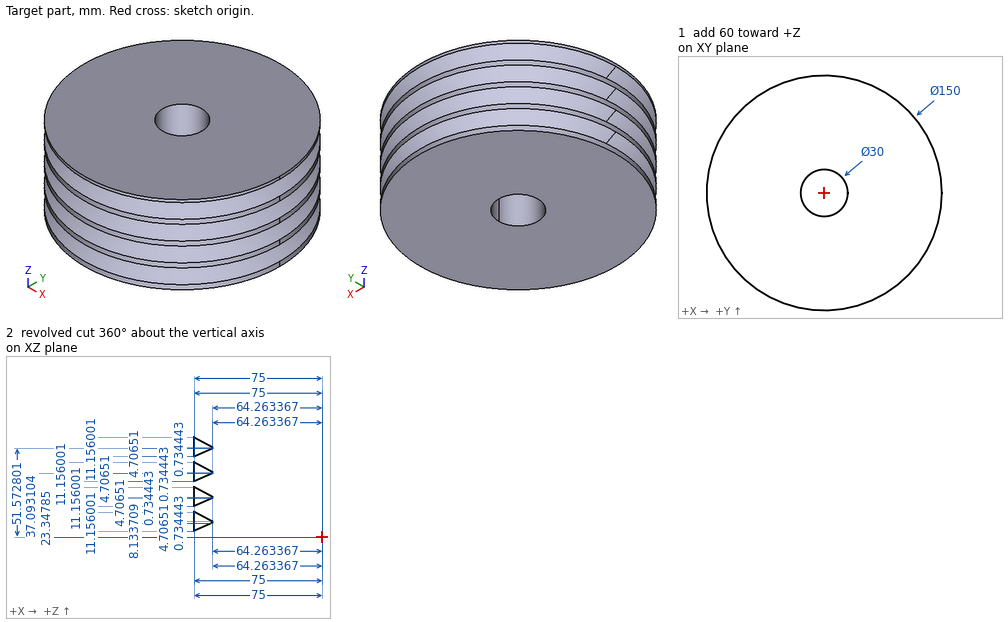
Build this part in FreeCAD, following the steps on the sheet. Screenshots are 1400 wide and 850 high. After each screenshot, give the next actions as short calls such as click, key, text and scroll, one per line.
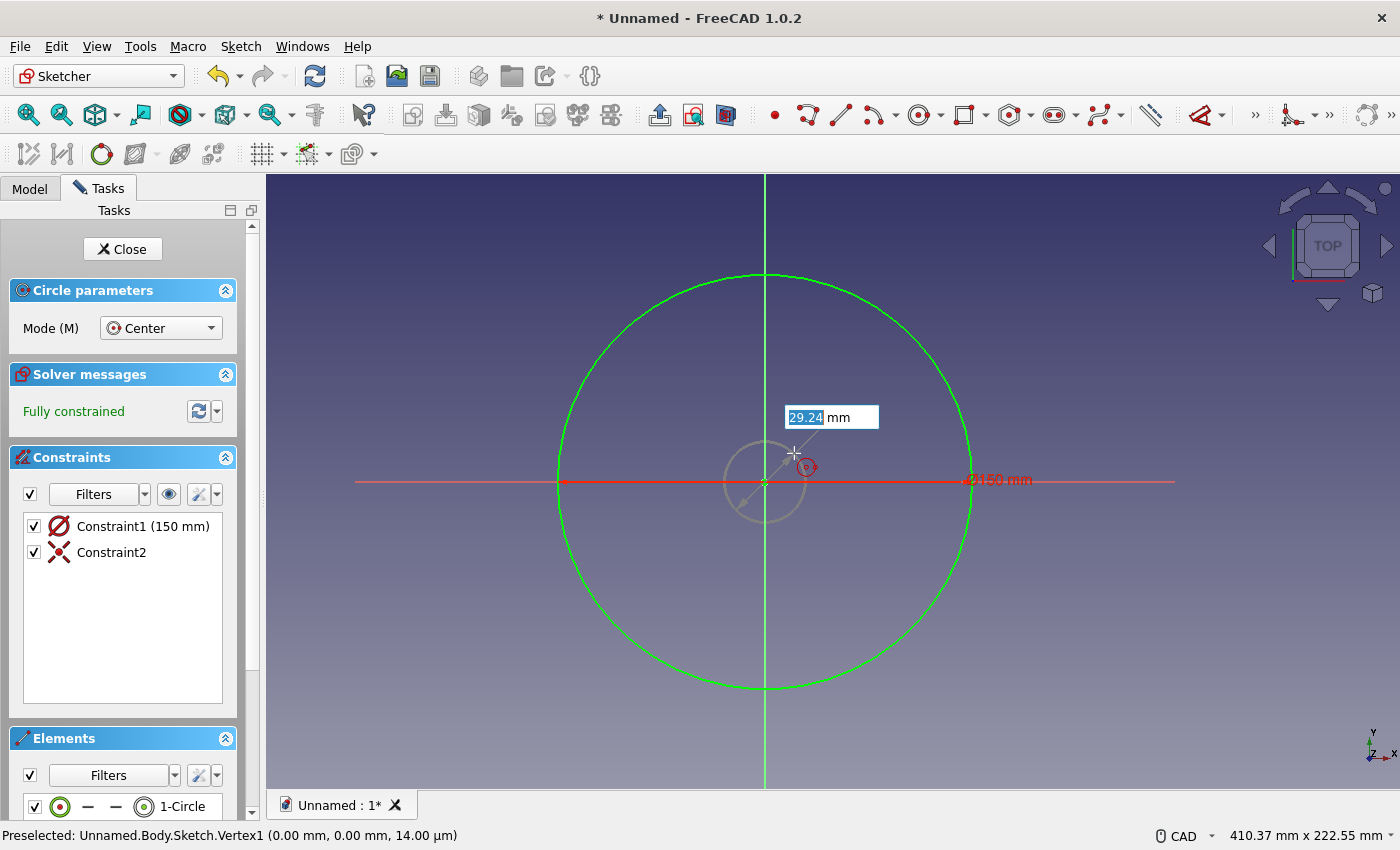
text(30)
key(Return)
key(Escape)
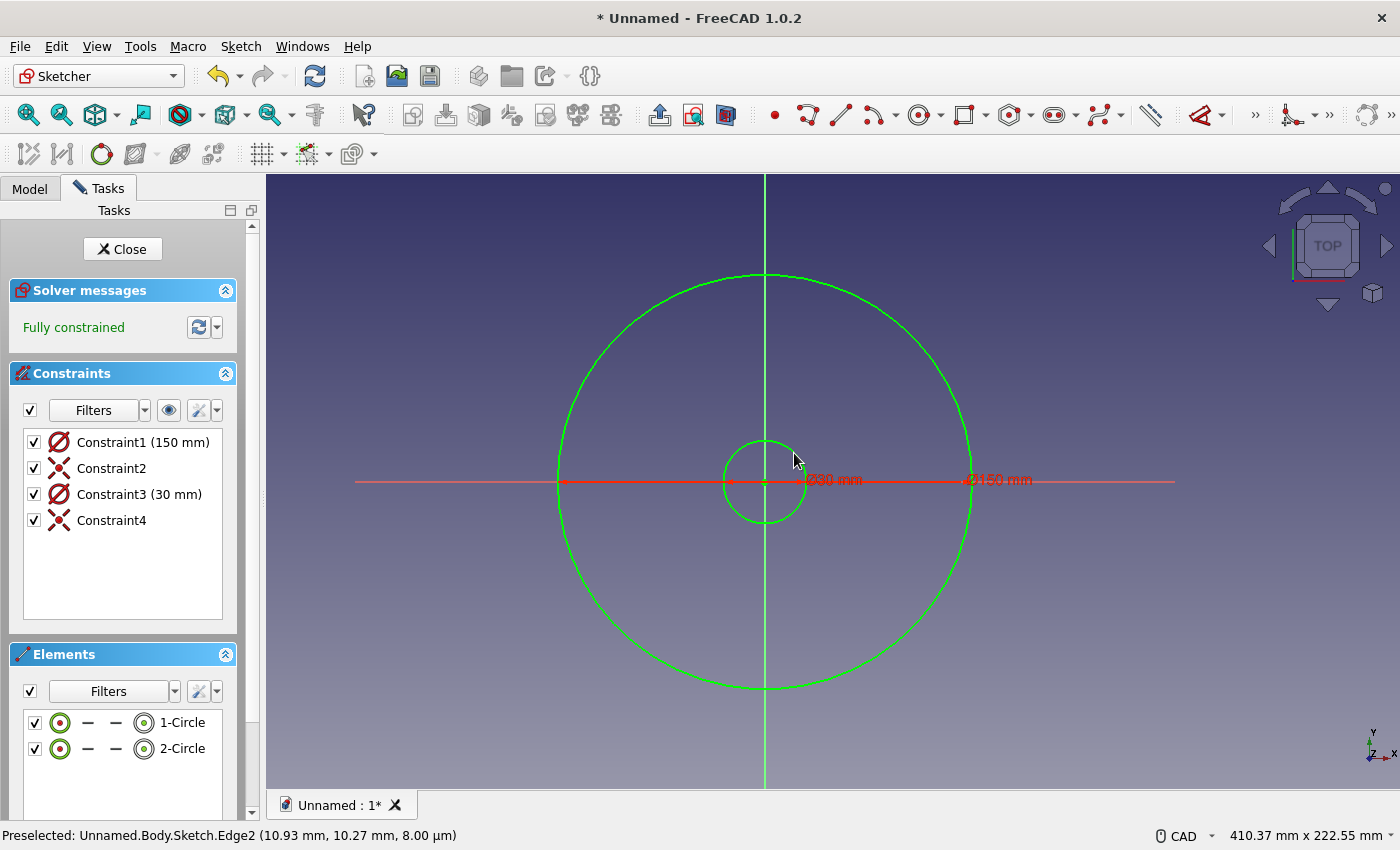
click(123, 249)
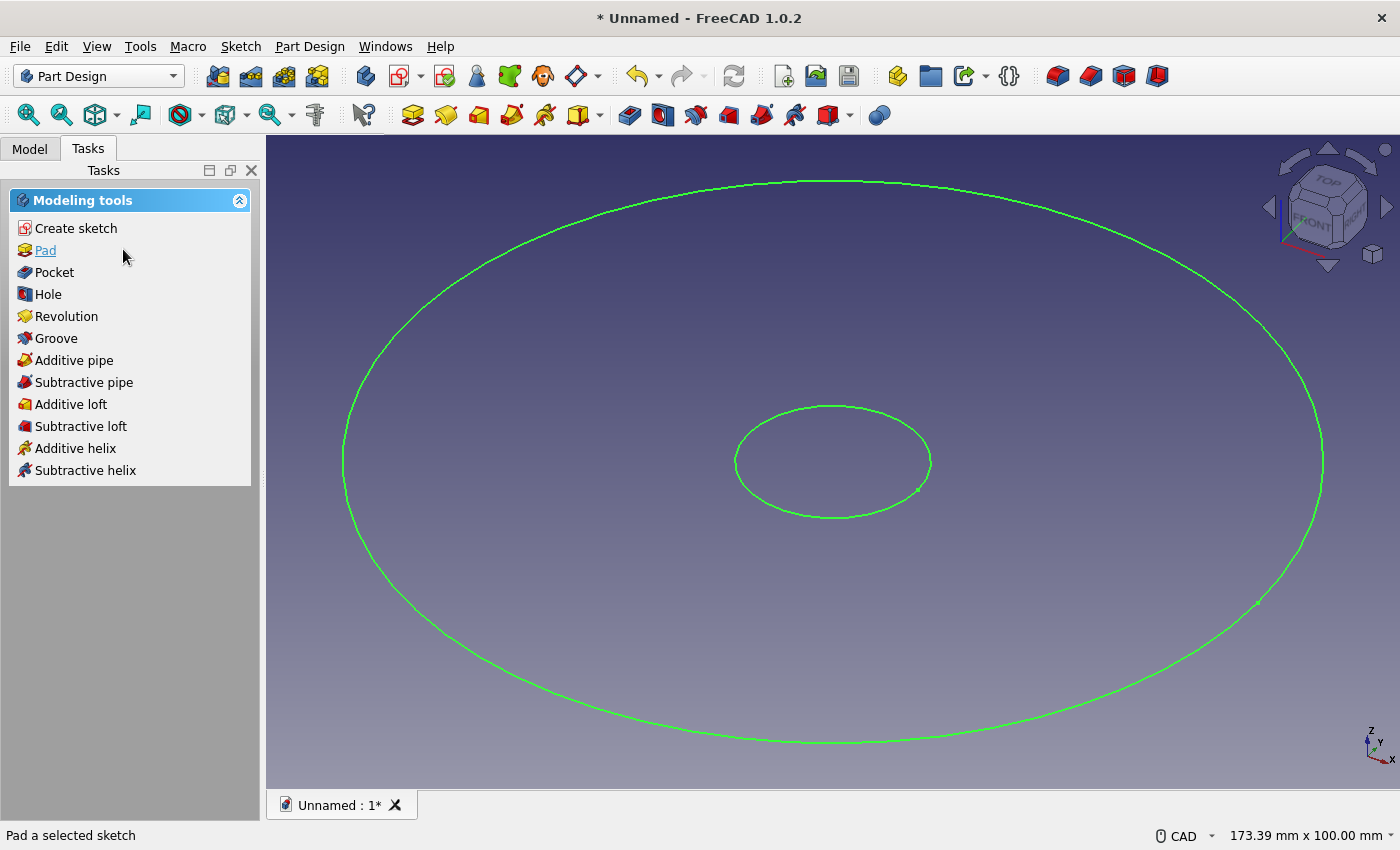
click(413, 116)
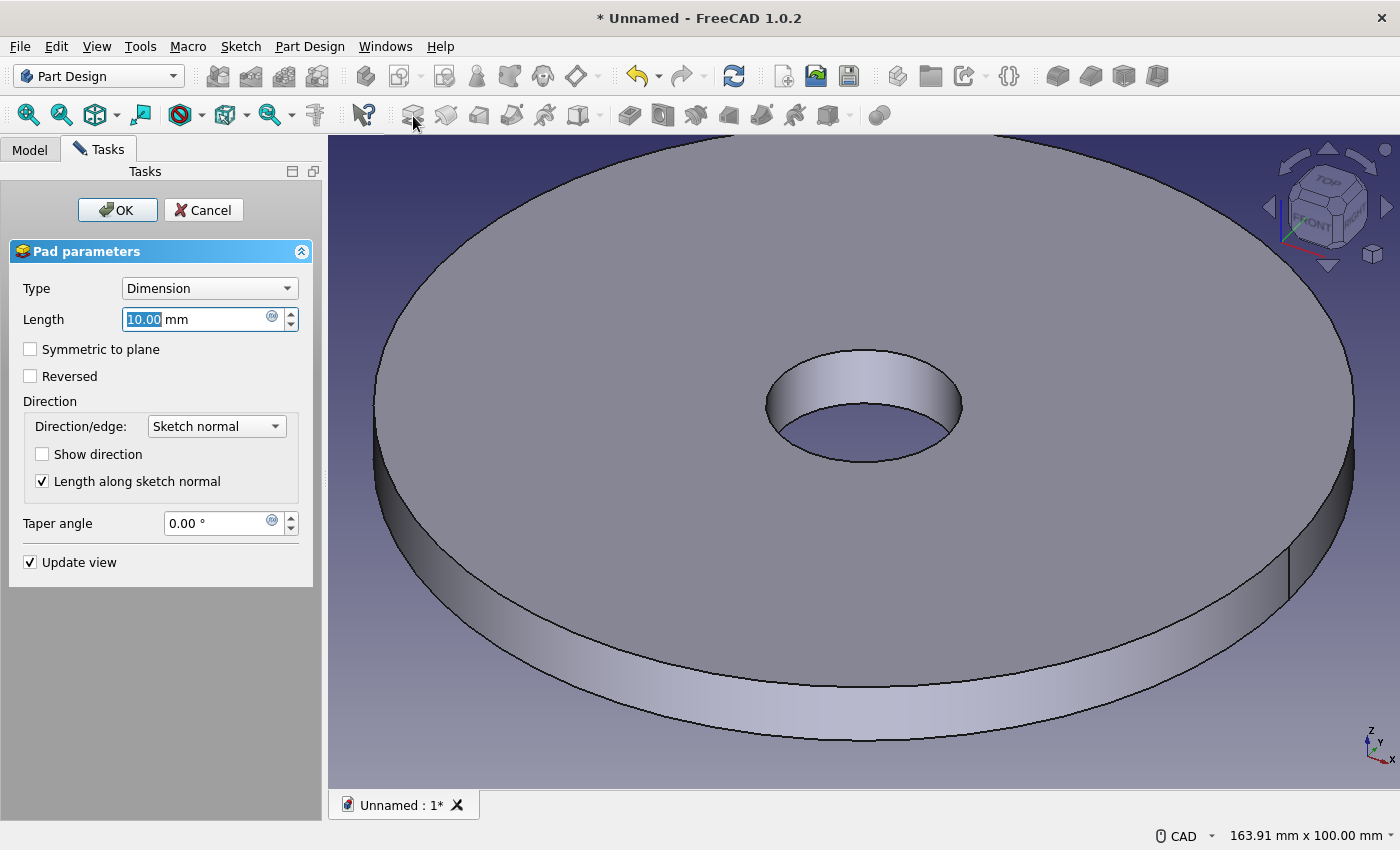
text(60)
key(Tab)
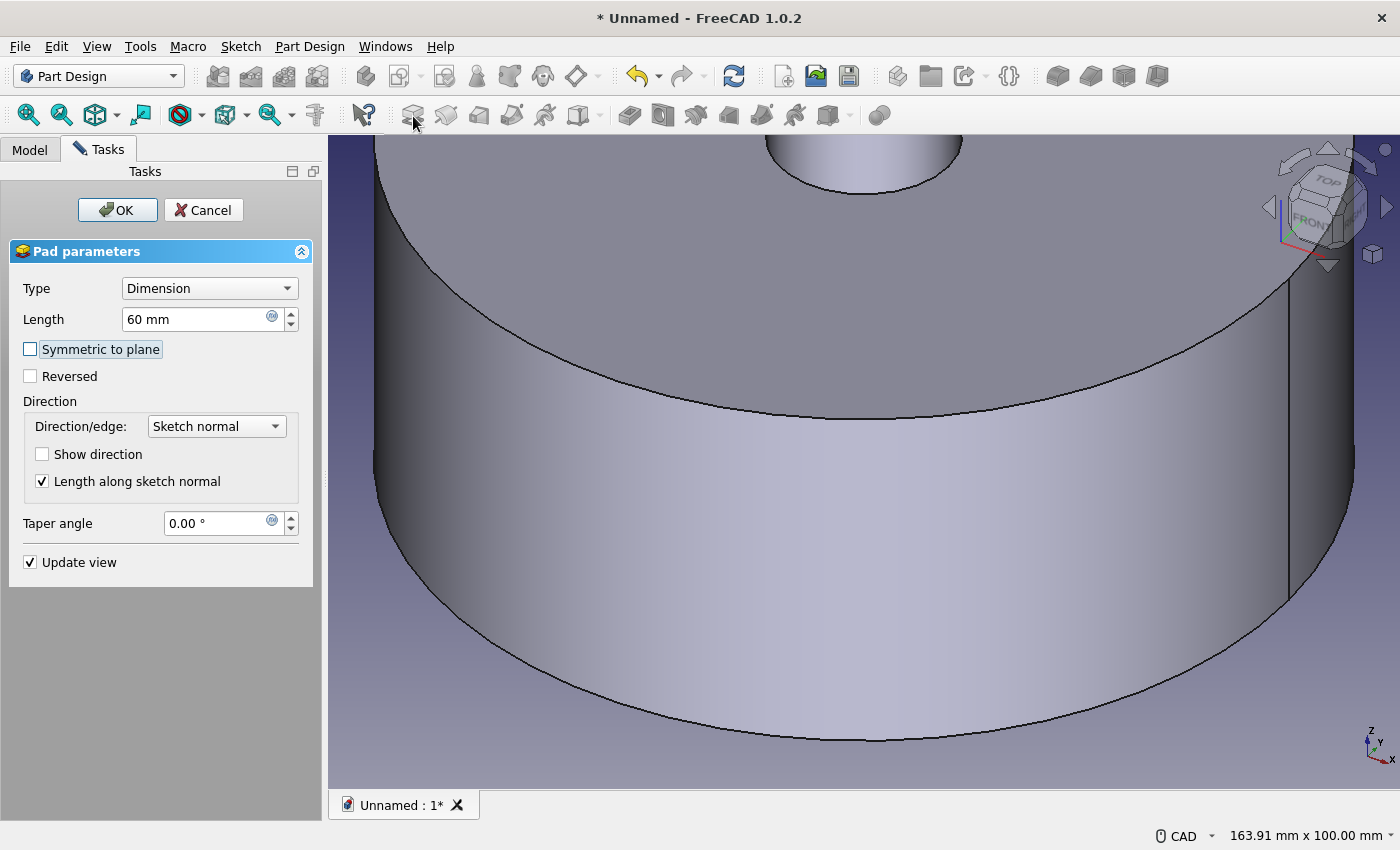
click(118, 210)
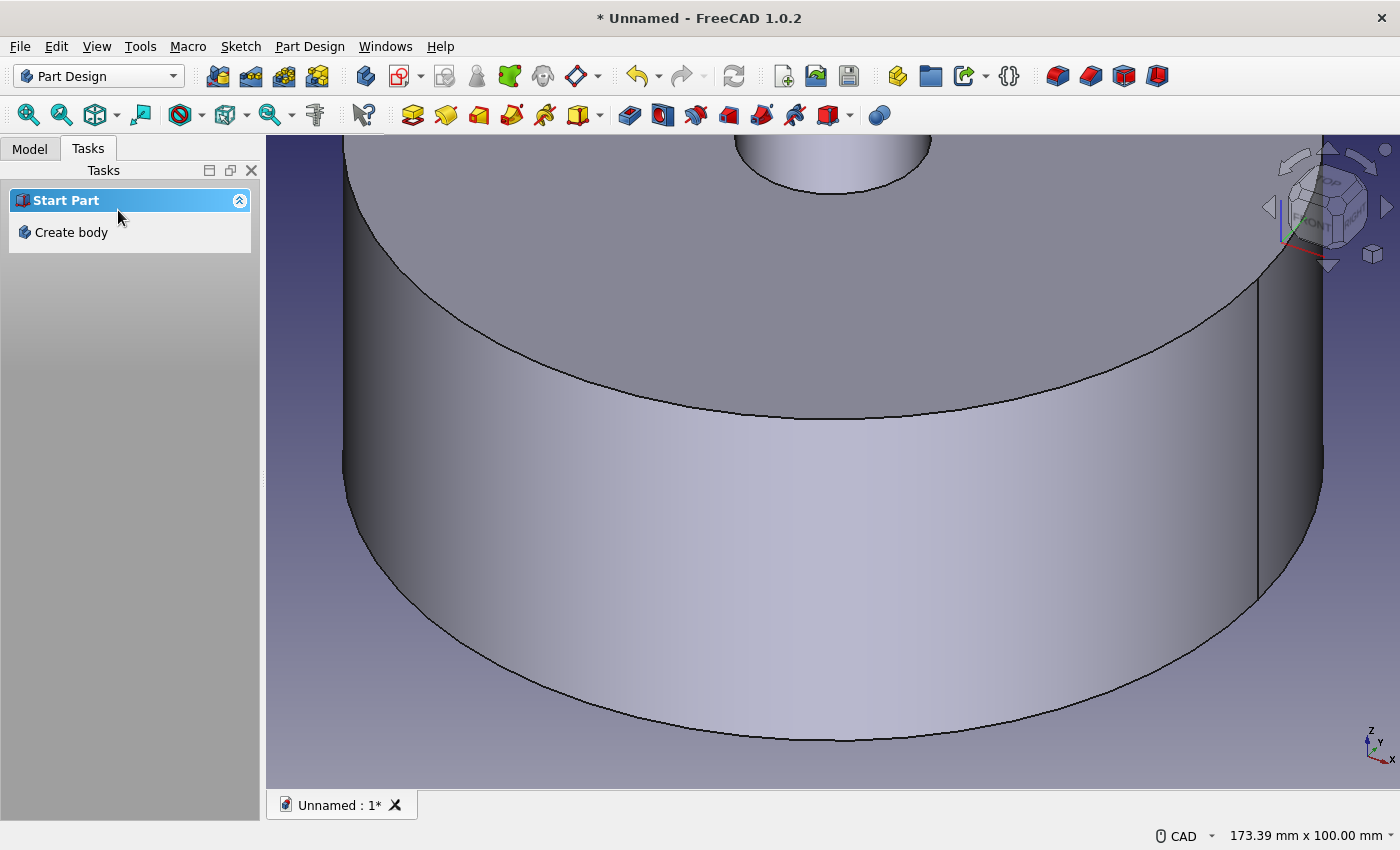
click(29, 116)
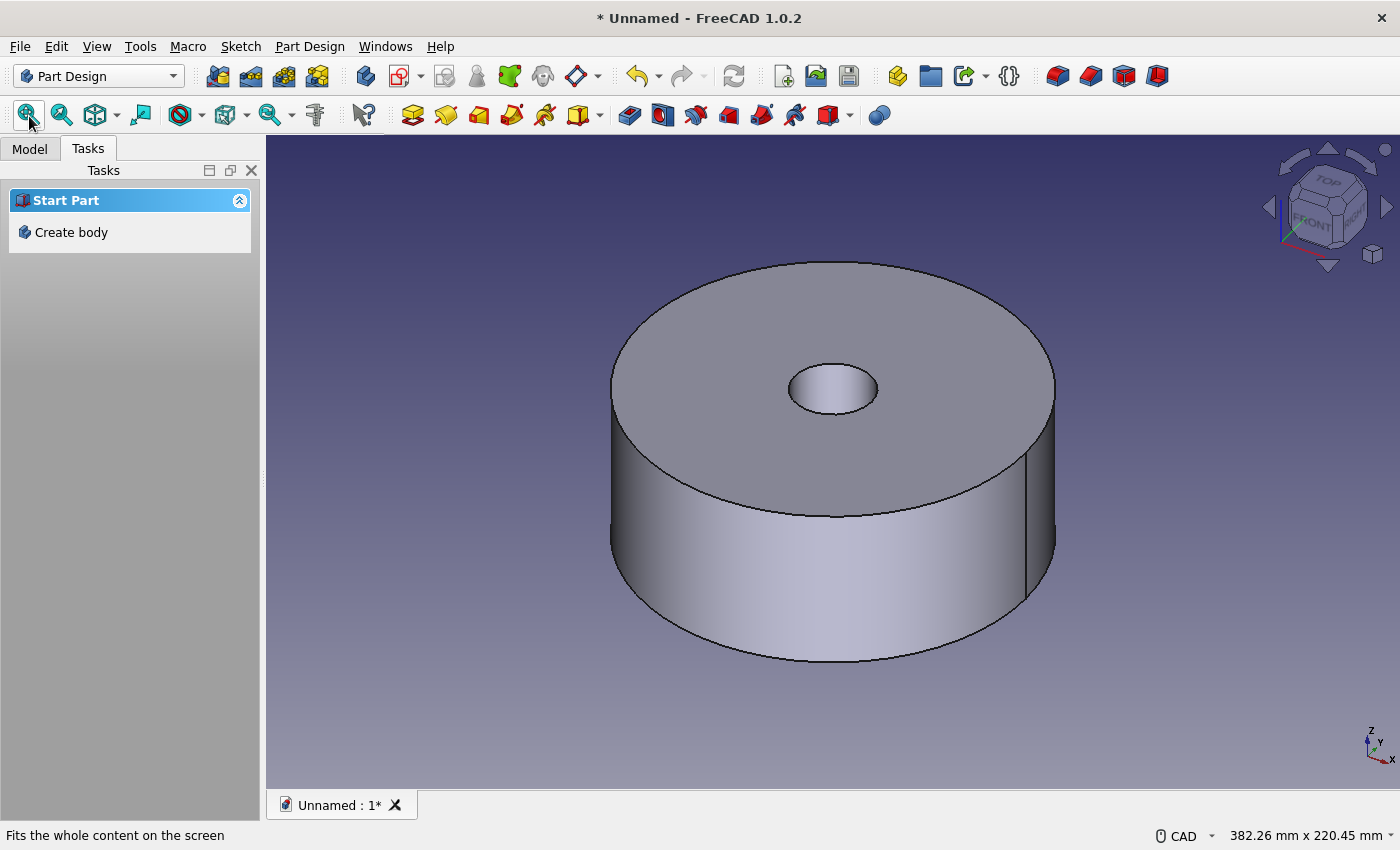
click(398, 76)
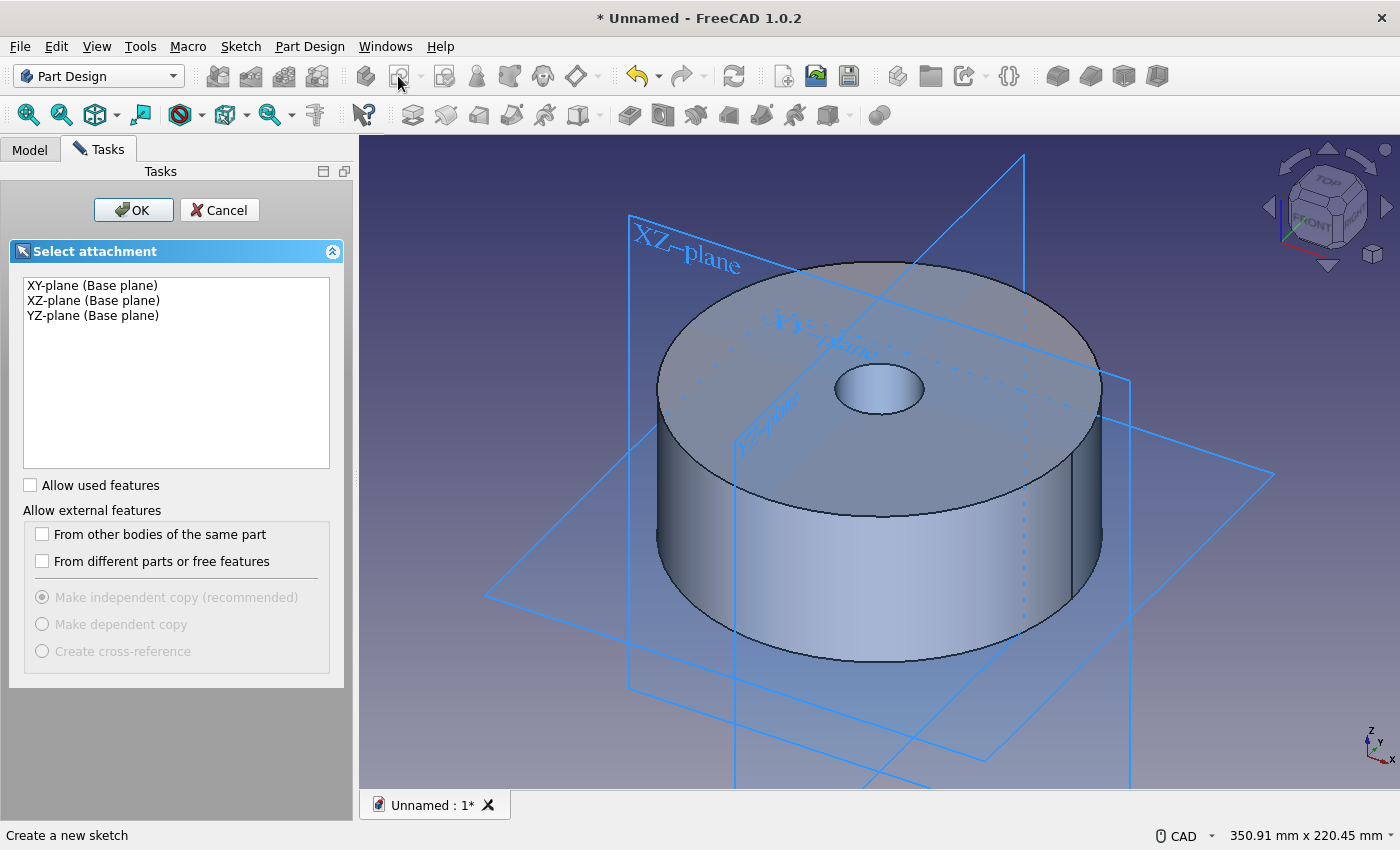
click(84, 300)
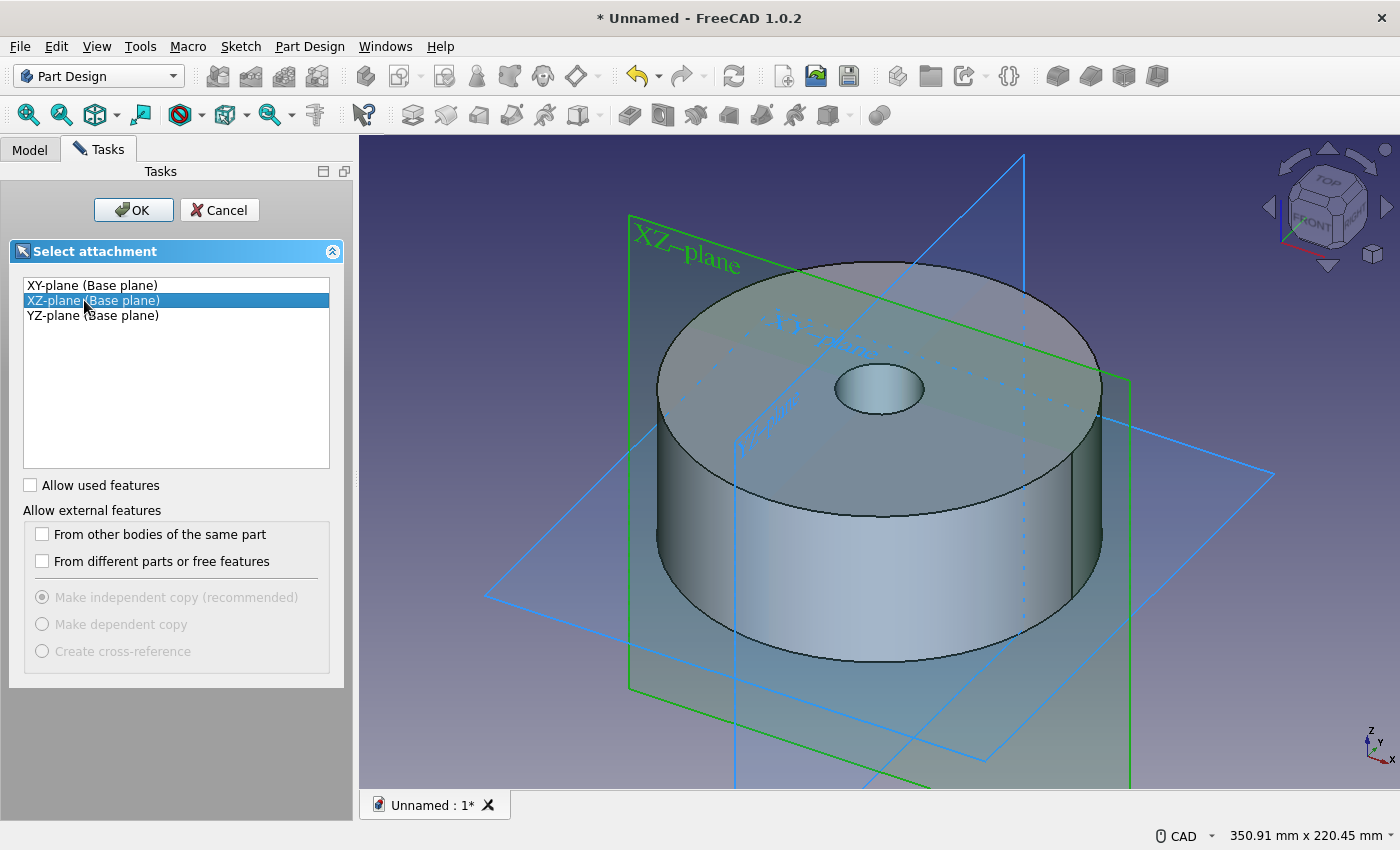
click(134, 210)